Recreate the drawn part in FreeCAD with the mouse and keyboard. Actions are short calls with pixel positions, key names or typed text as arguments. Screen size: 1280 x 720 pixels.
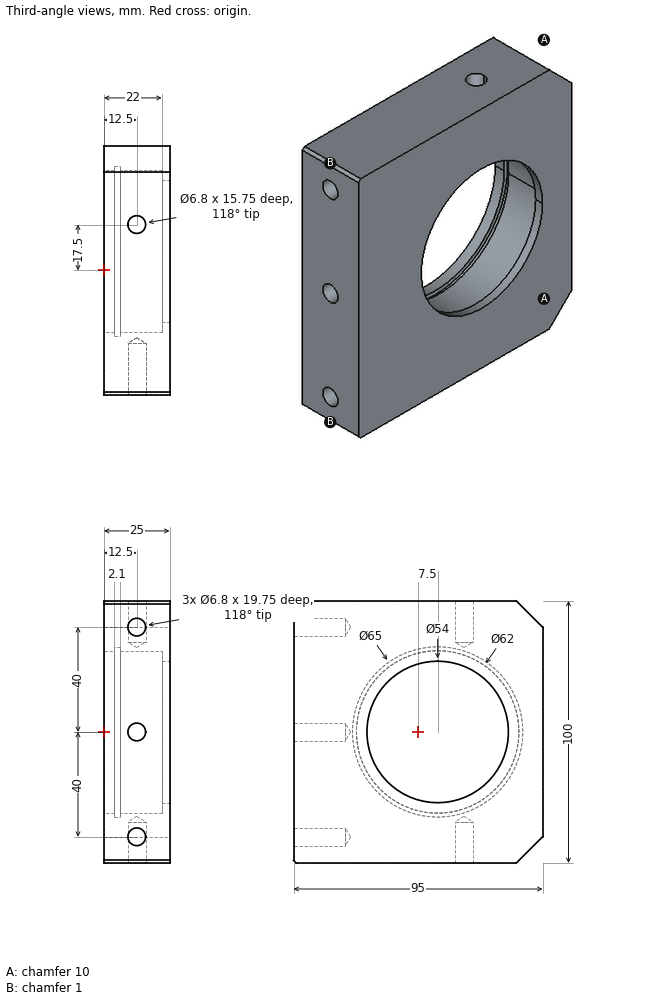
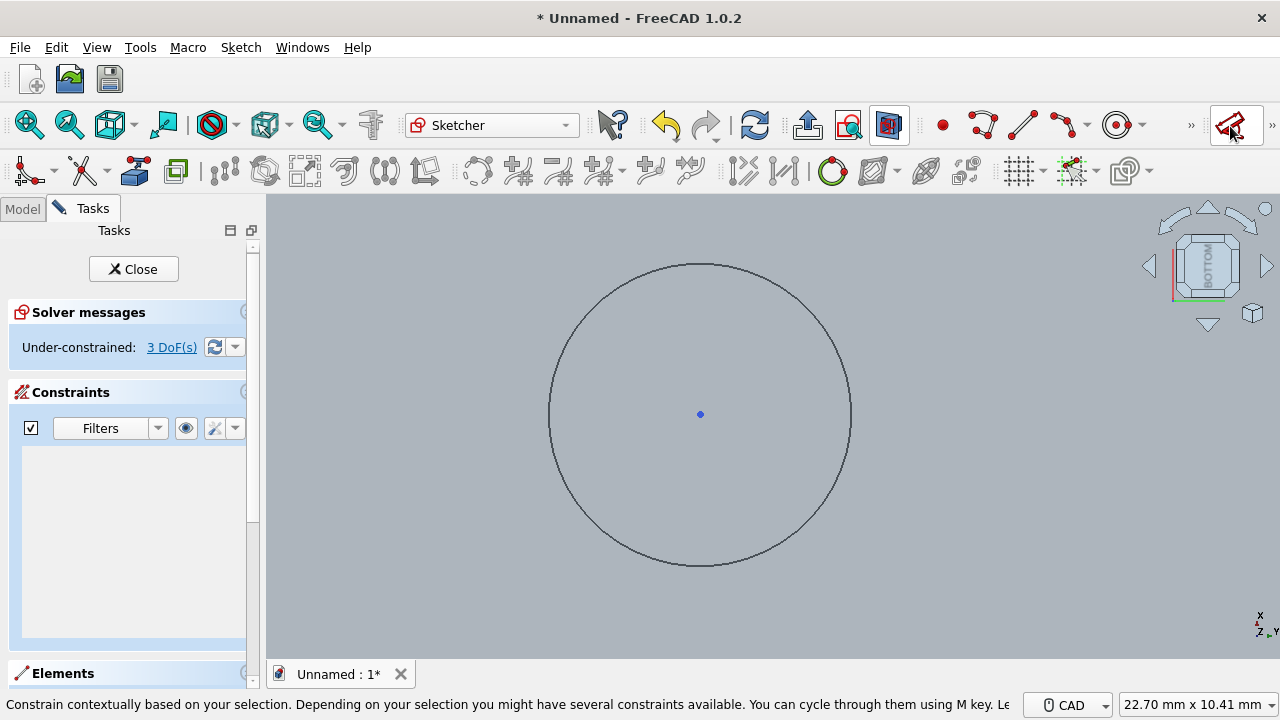
click(807, 308)
click(830, 285)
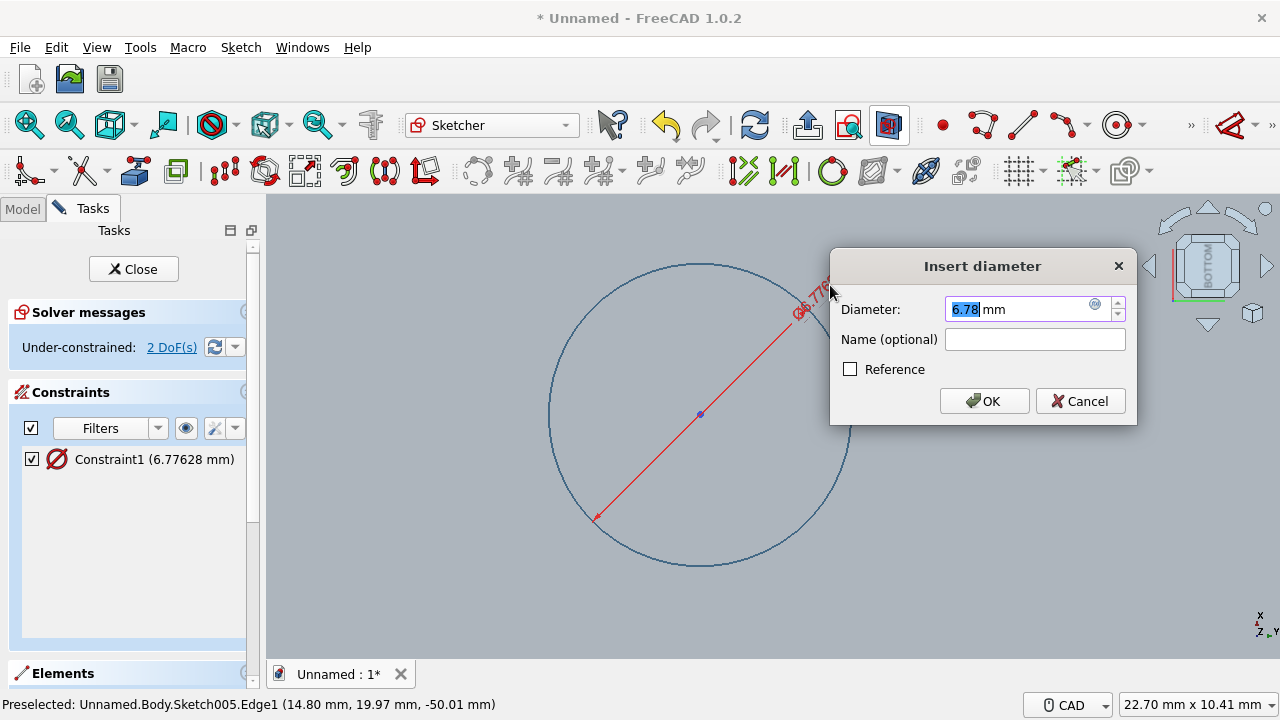
text(6.8)
key(Return)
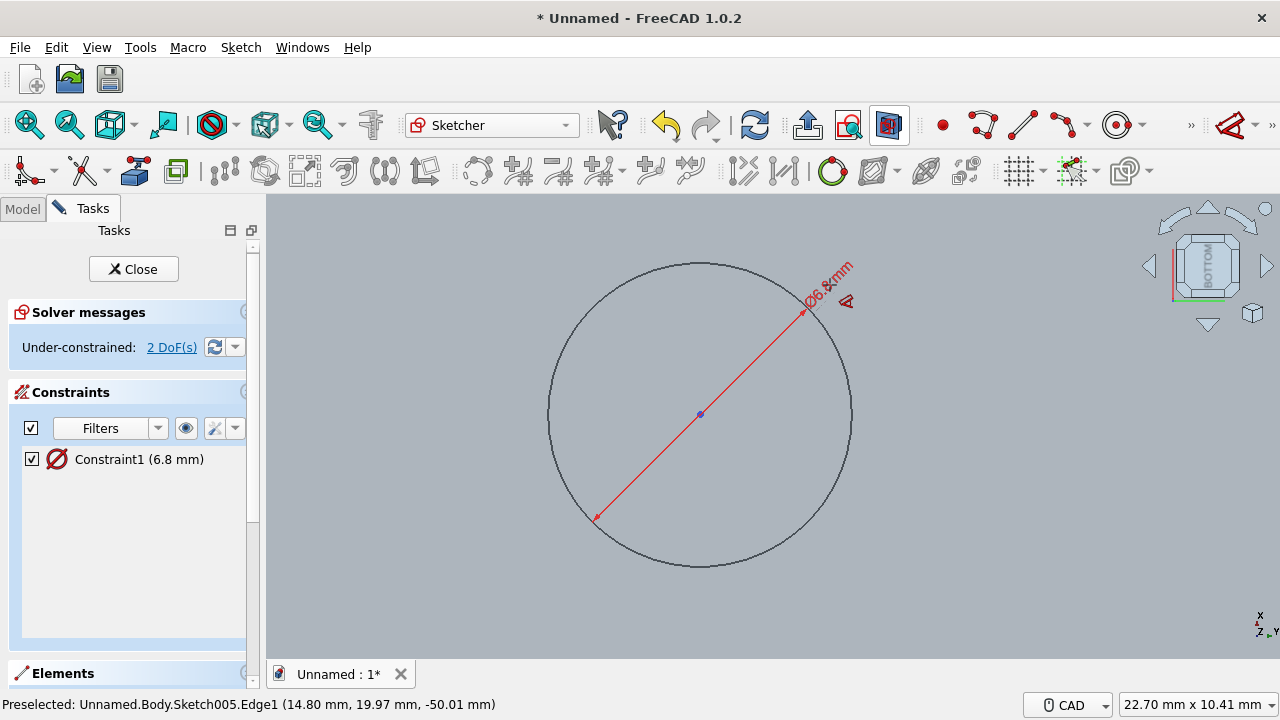
click(700, 415)
click(497, 381)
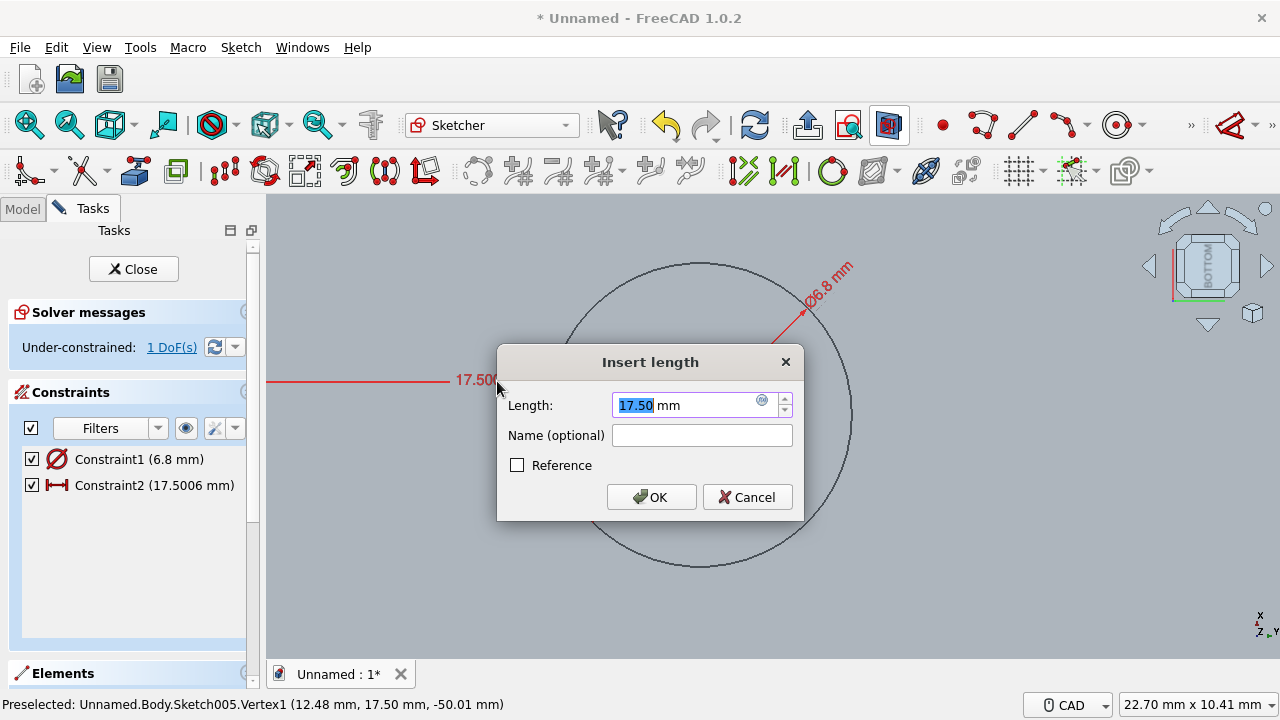
text(17.5)
key(Return)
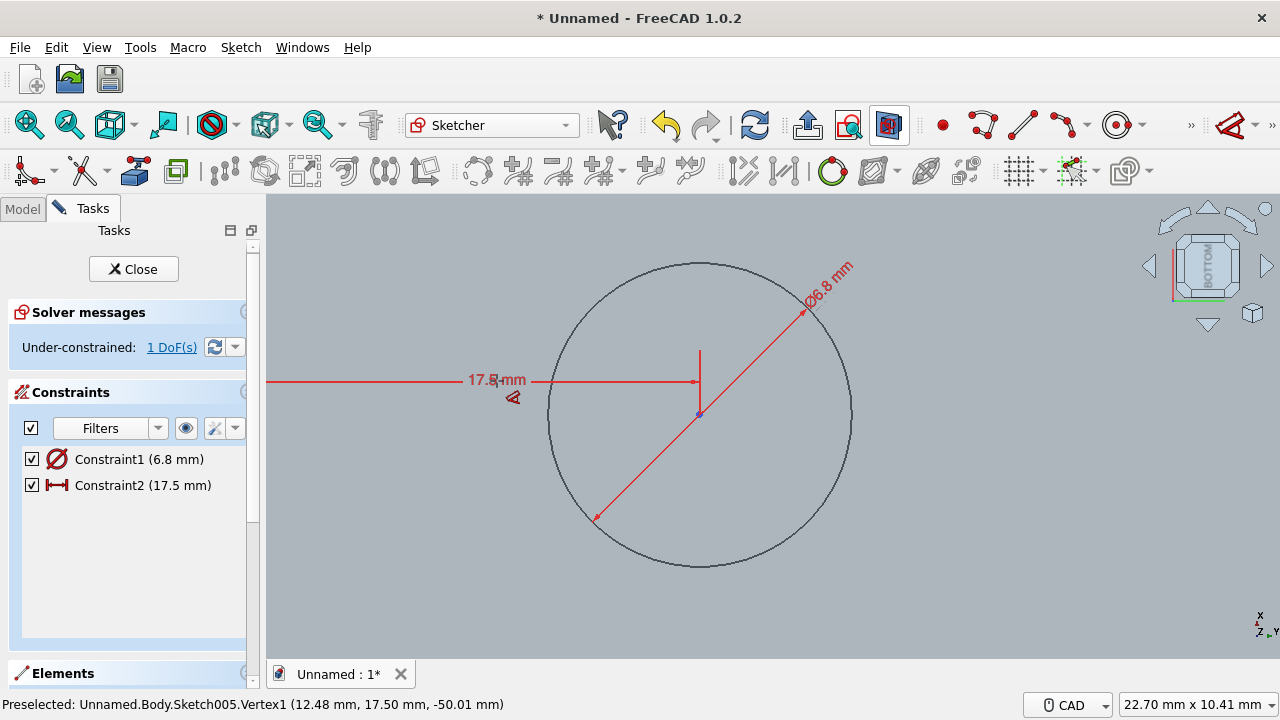
click(700, 415)
click(734, 523)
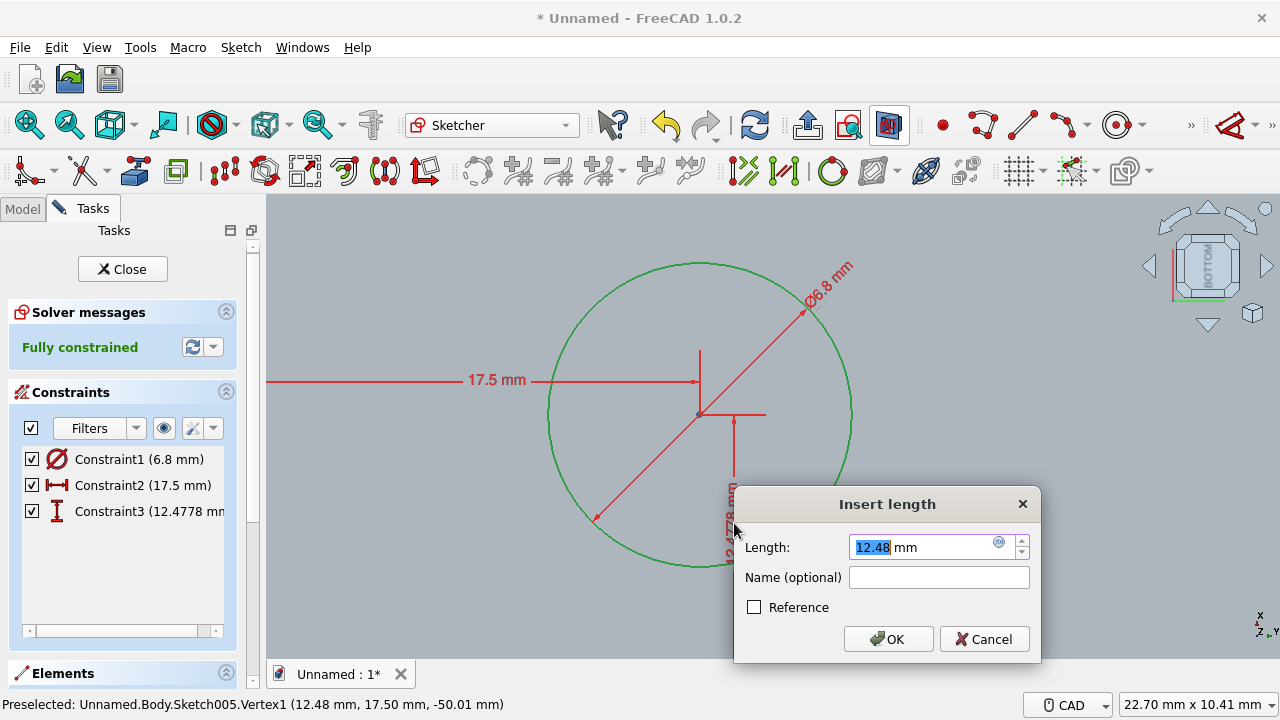
text(12.5)
key(Return)
key(Escape)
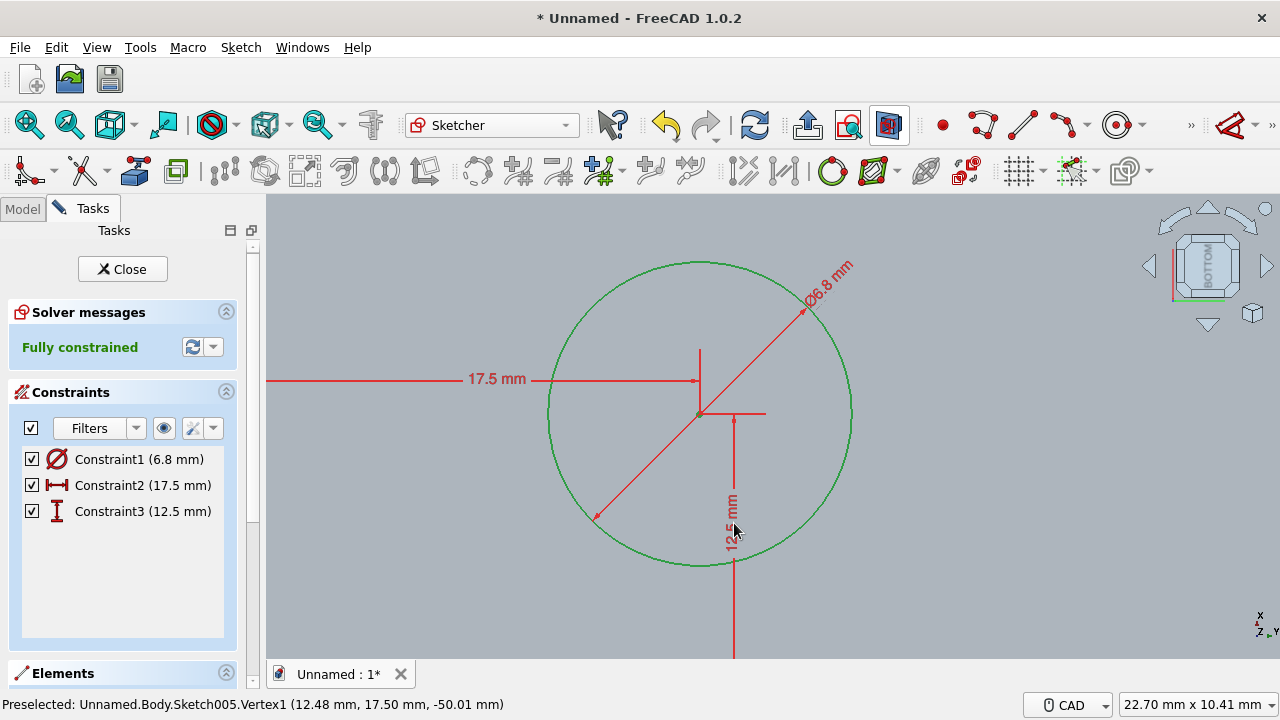
click(123, 269)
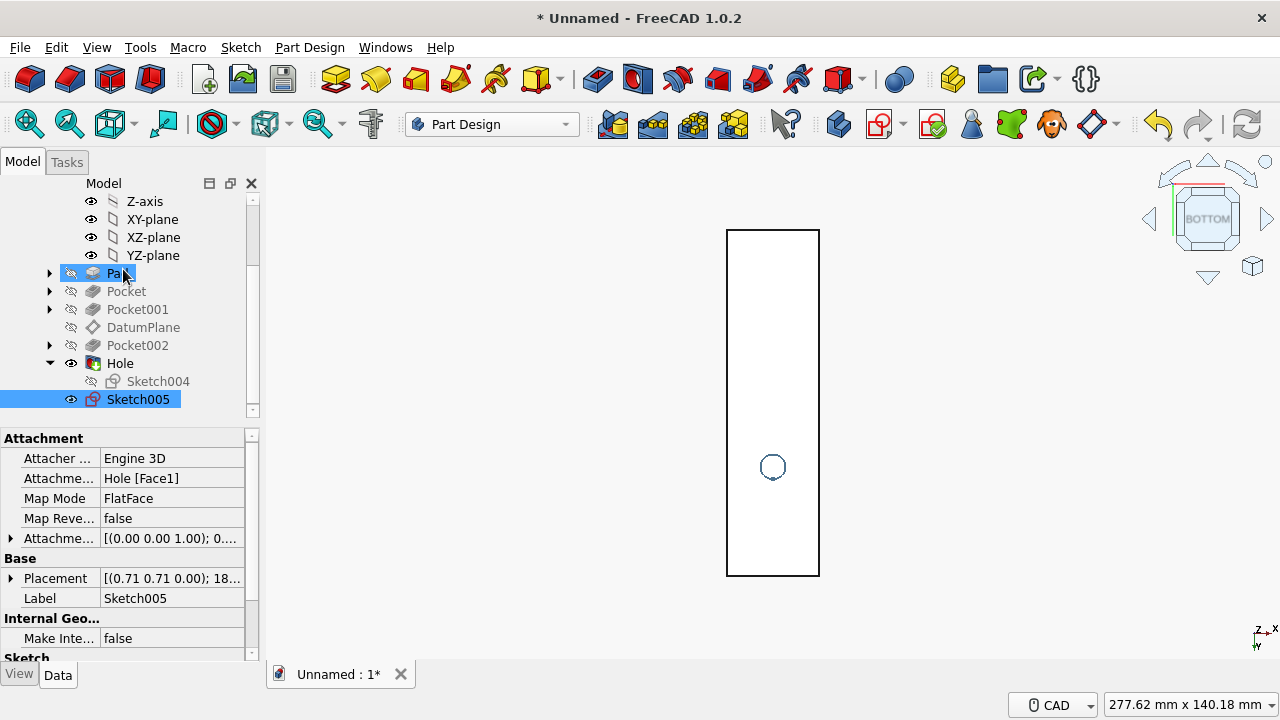
click(638, 80)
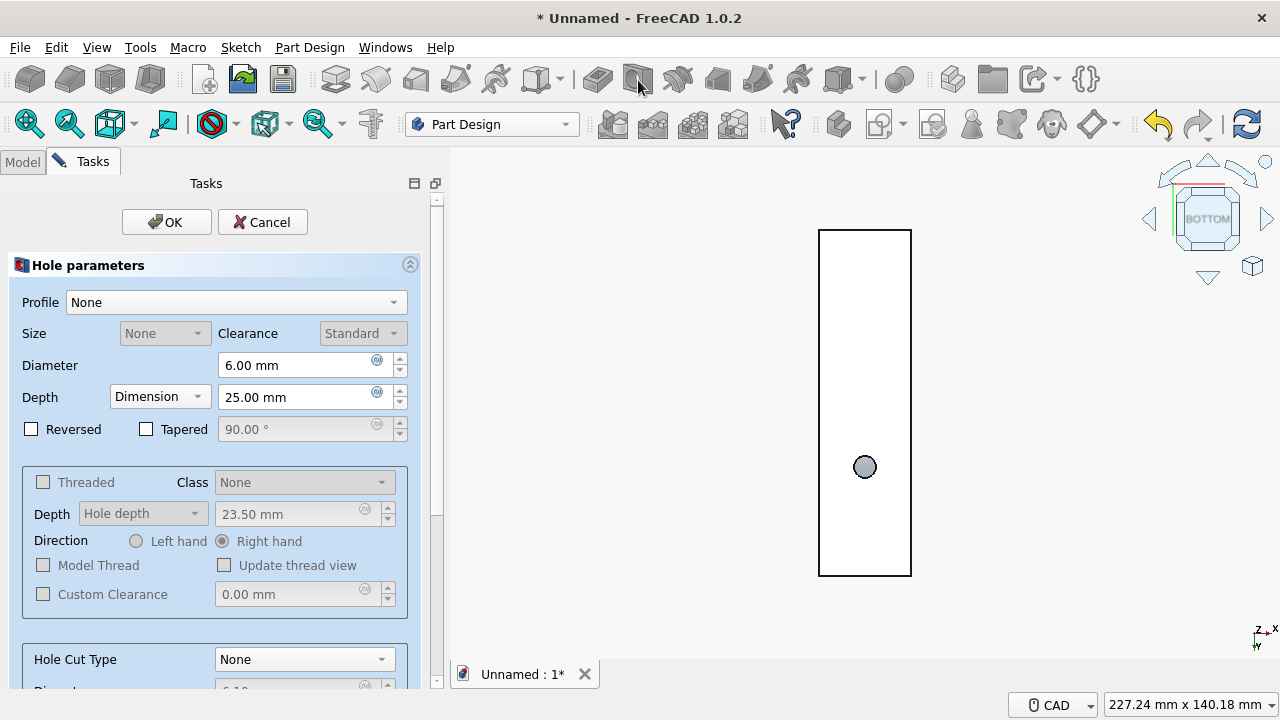
triple_click(305, 365)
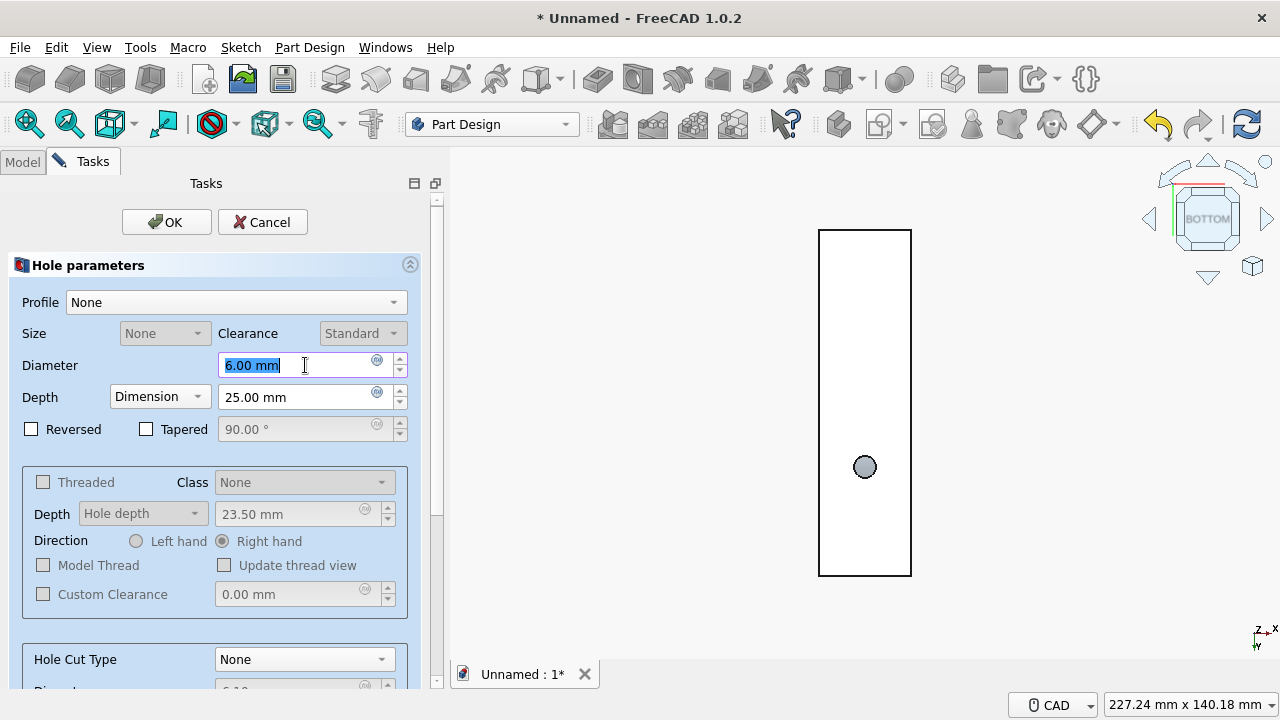
text(6.8)
key(Tab)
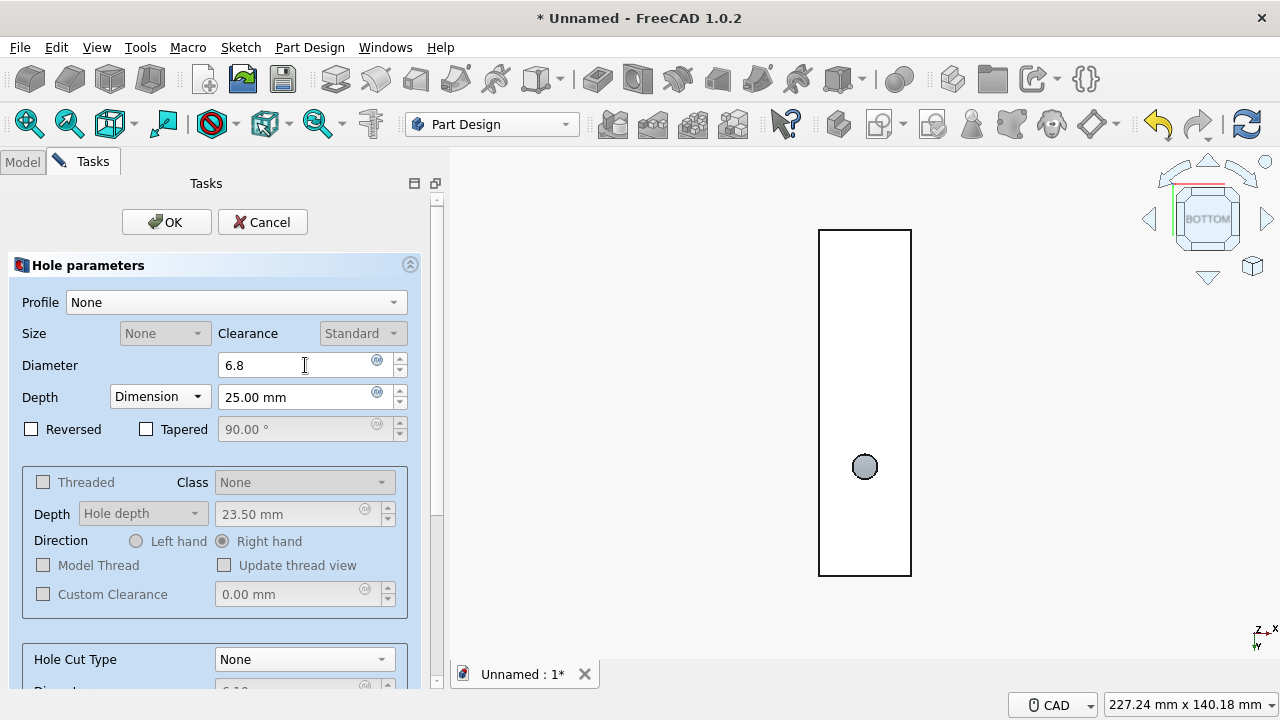
triple_click(305, 397)